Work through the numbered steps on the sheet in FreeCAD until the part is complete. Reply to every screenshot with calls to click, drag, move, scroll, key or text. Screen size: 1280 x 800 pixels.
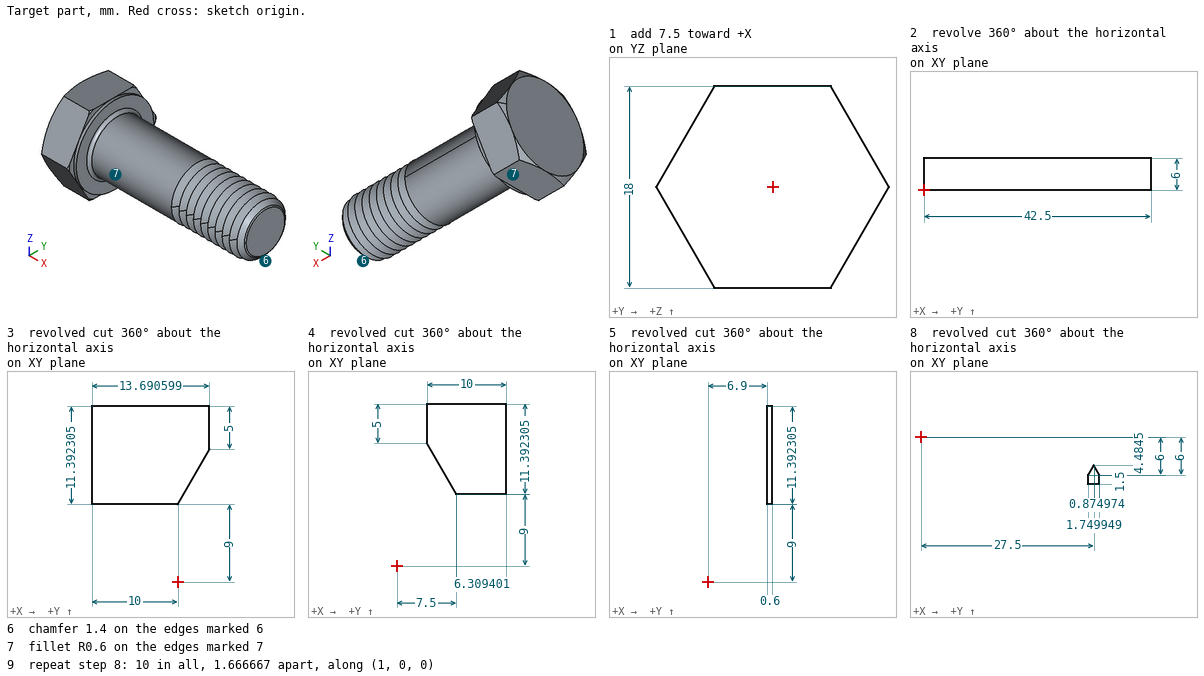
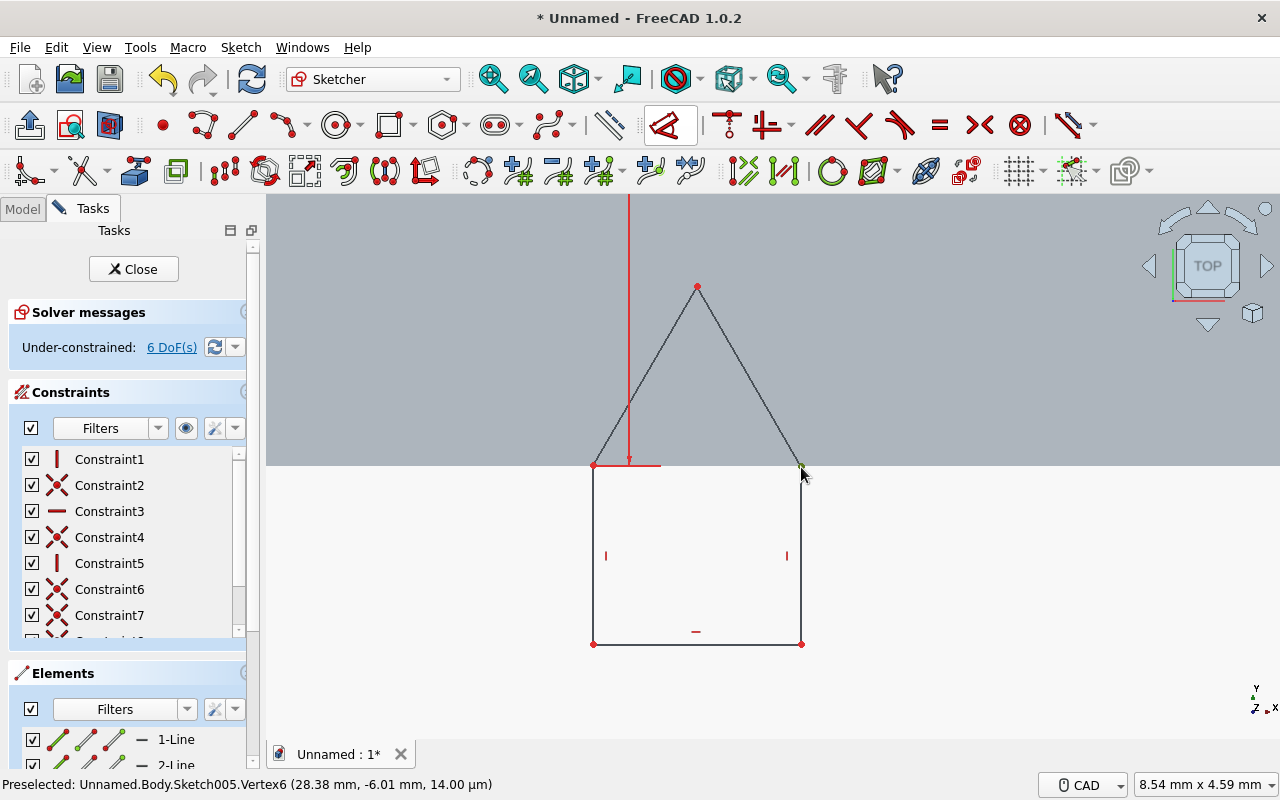
key(i)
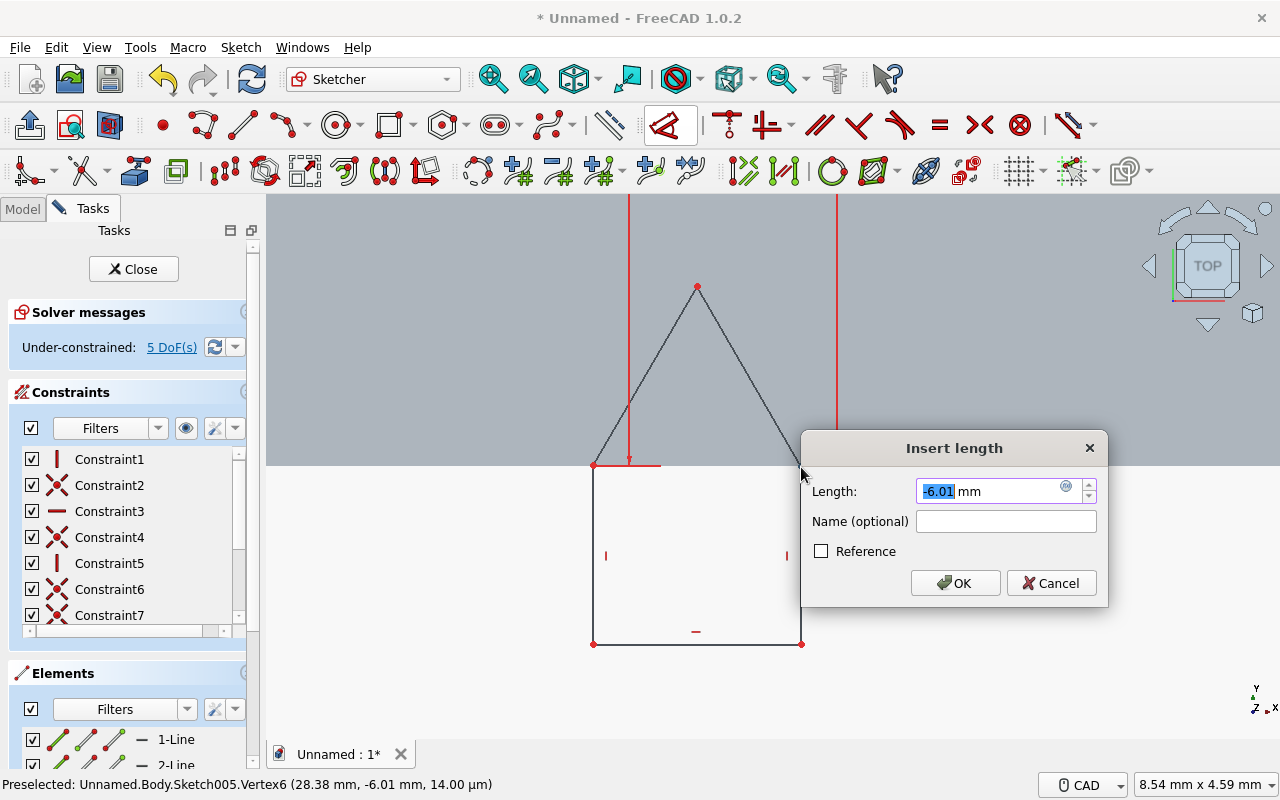
text(-6)
key(Return)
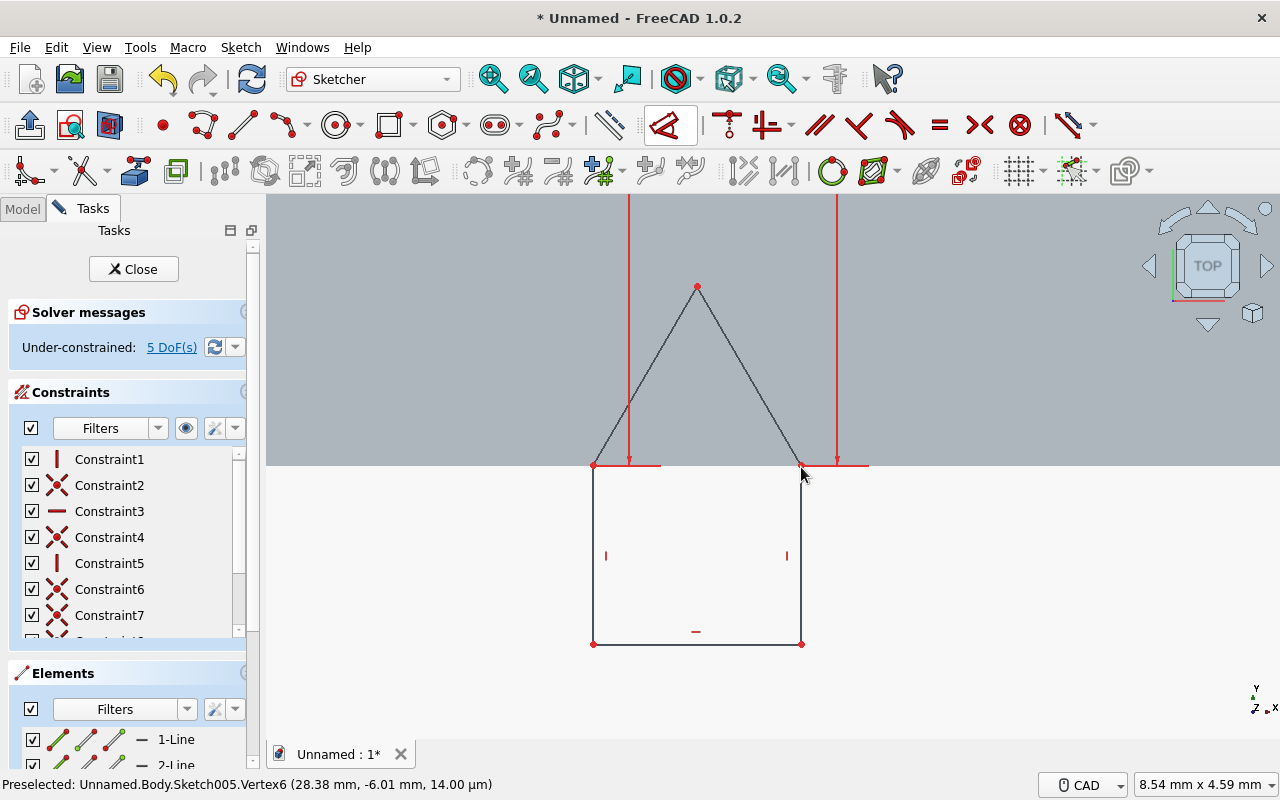
click(593, 519)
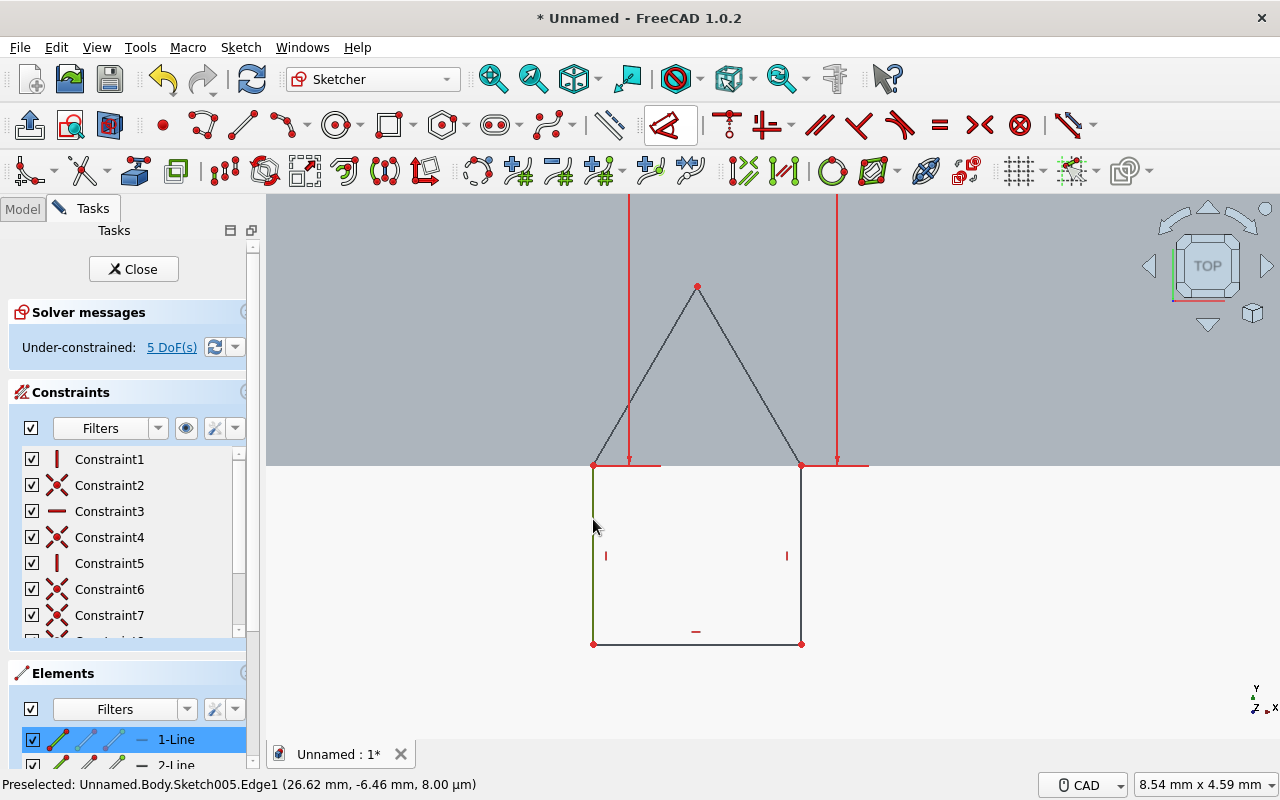
key(i)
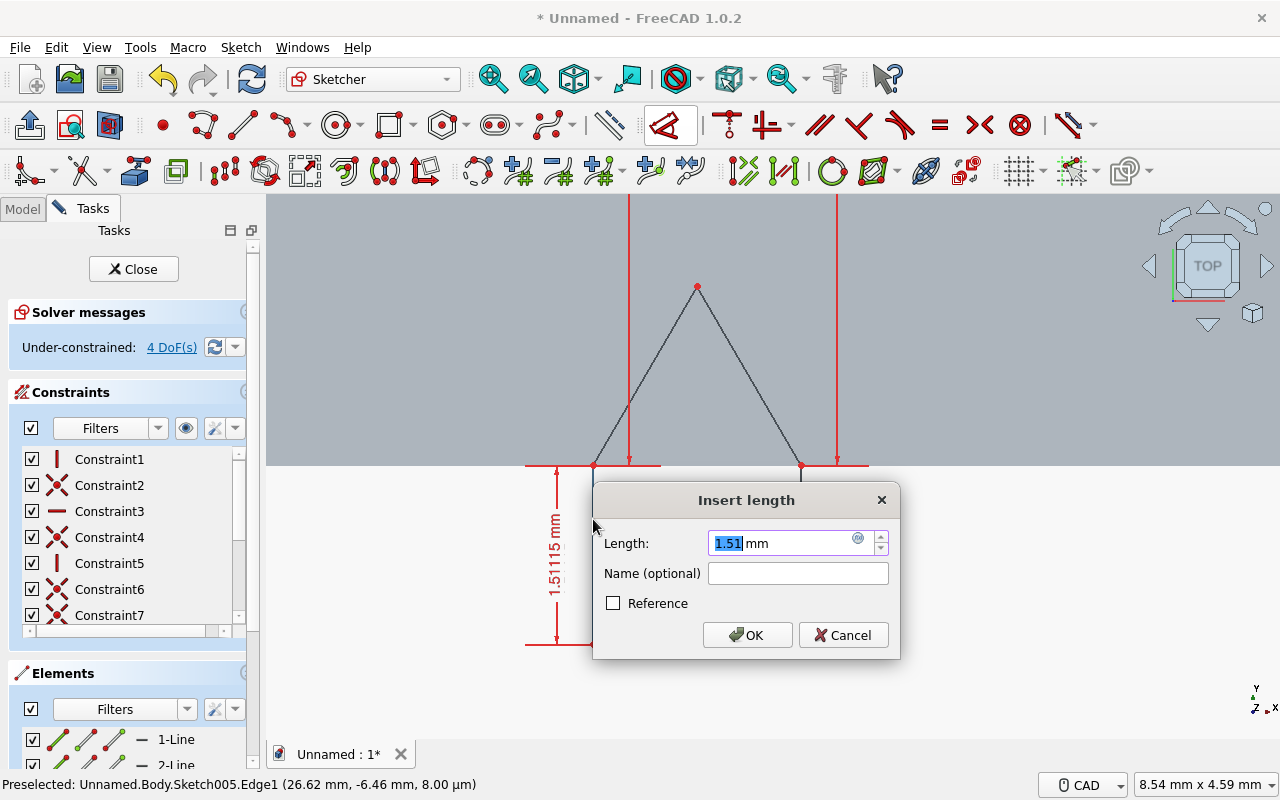
text(1.5)
key(Return)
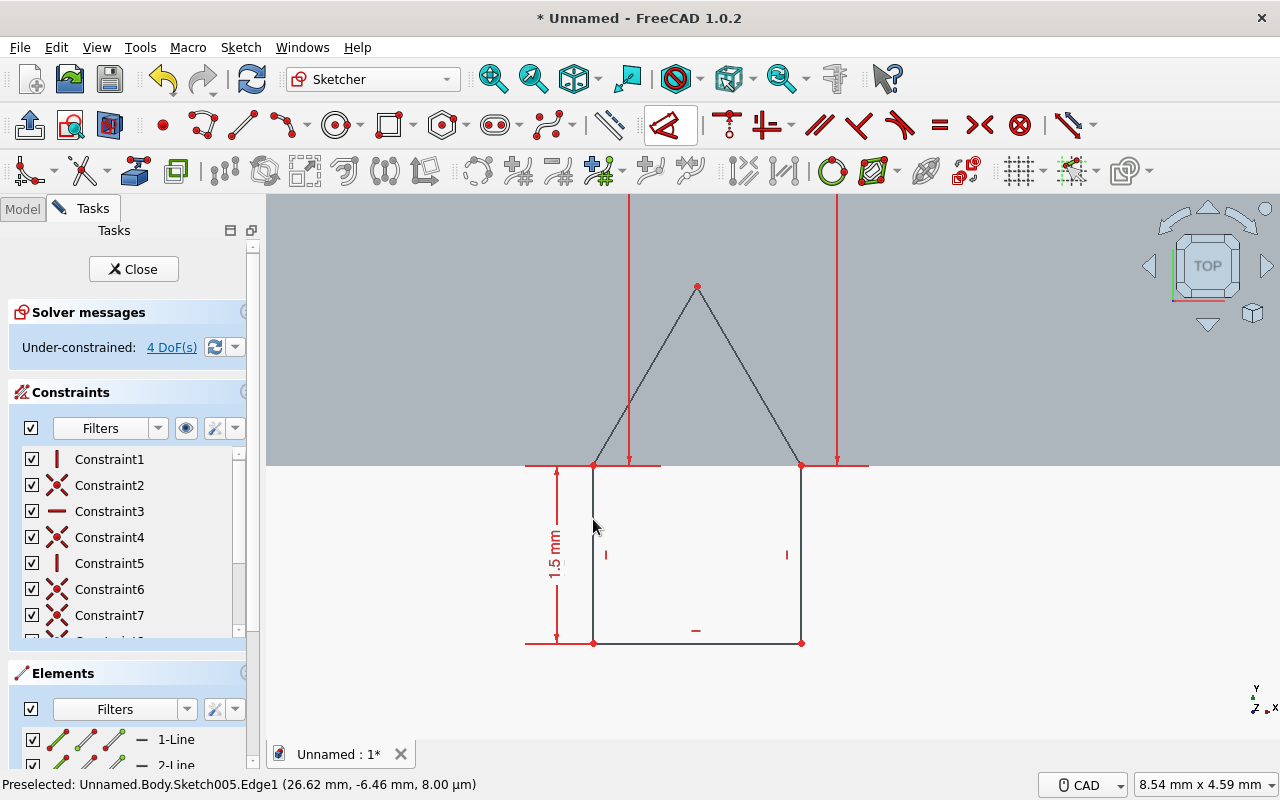
click(697, 287)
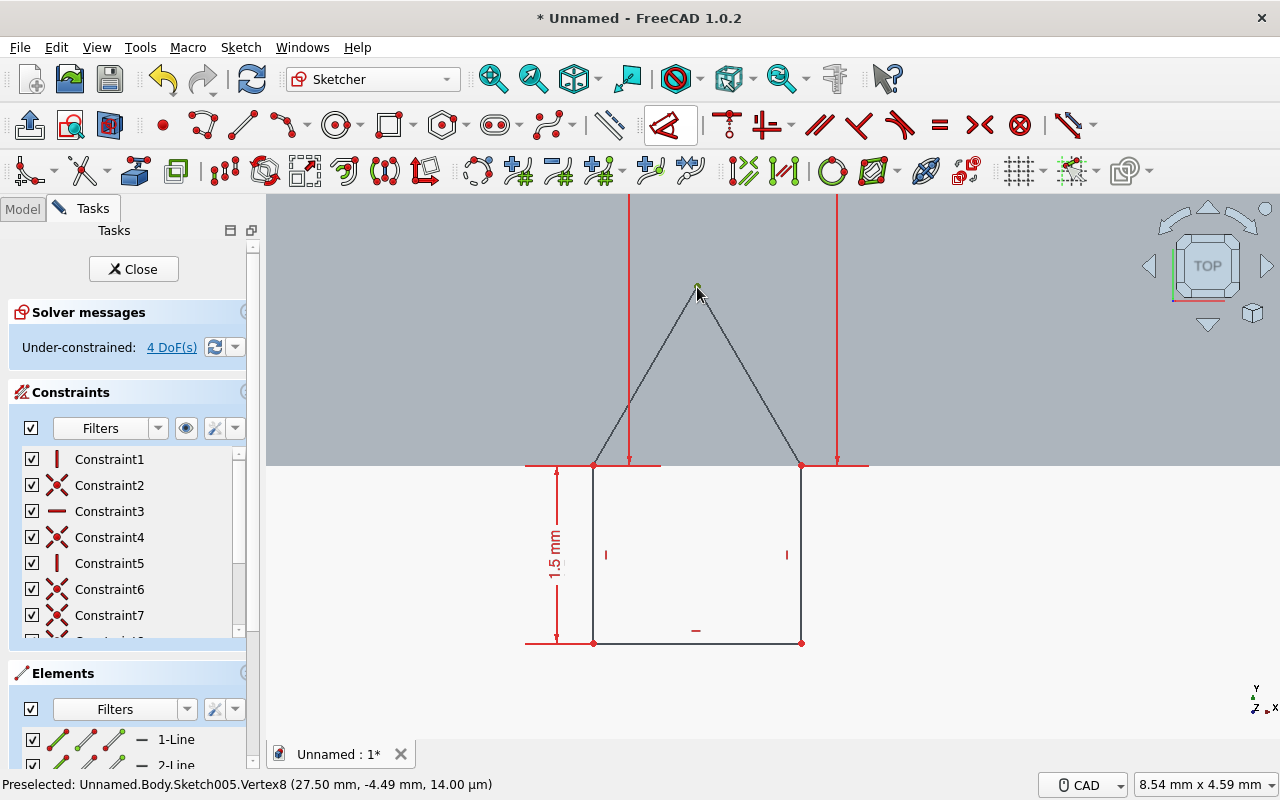
click(692, 126)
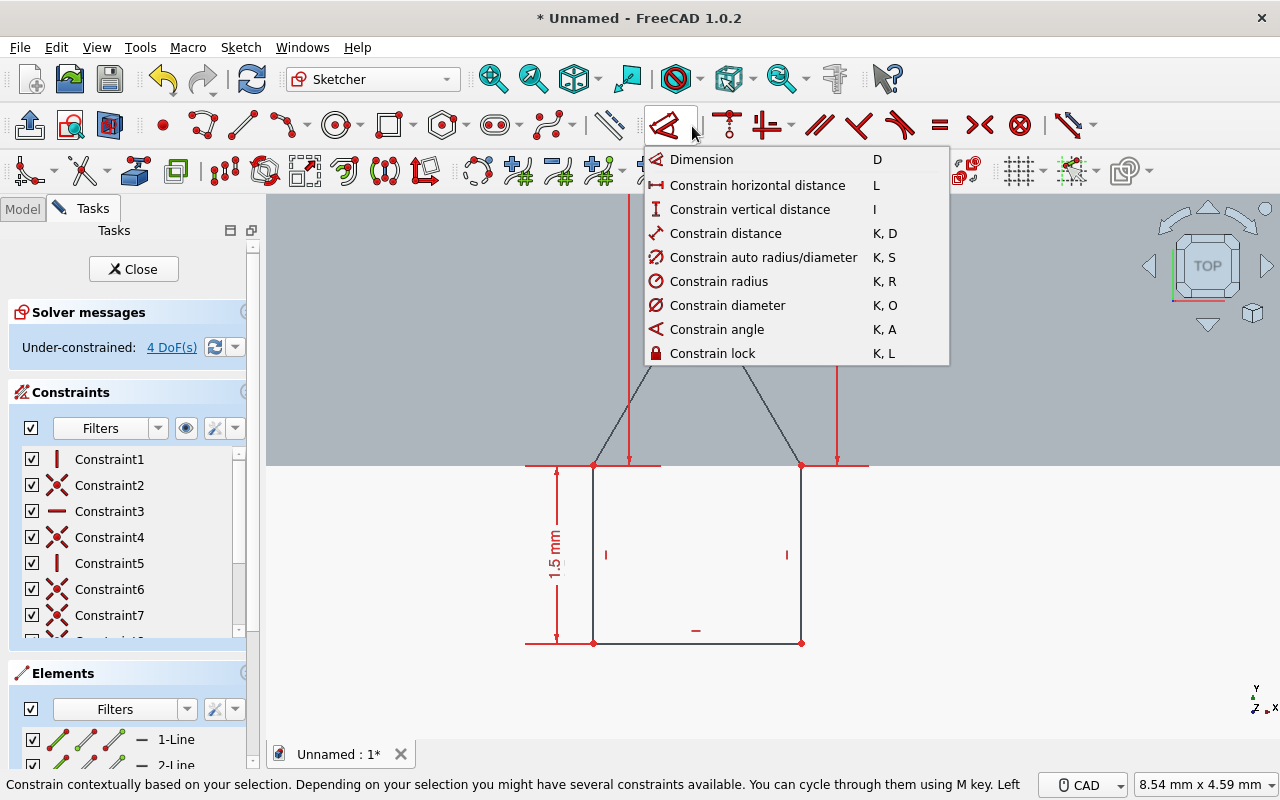
click(797, 185)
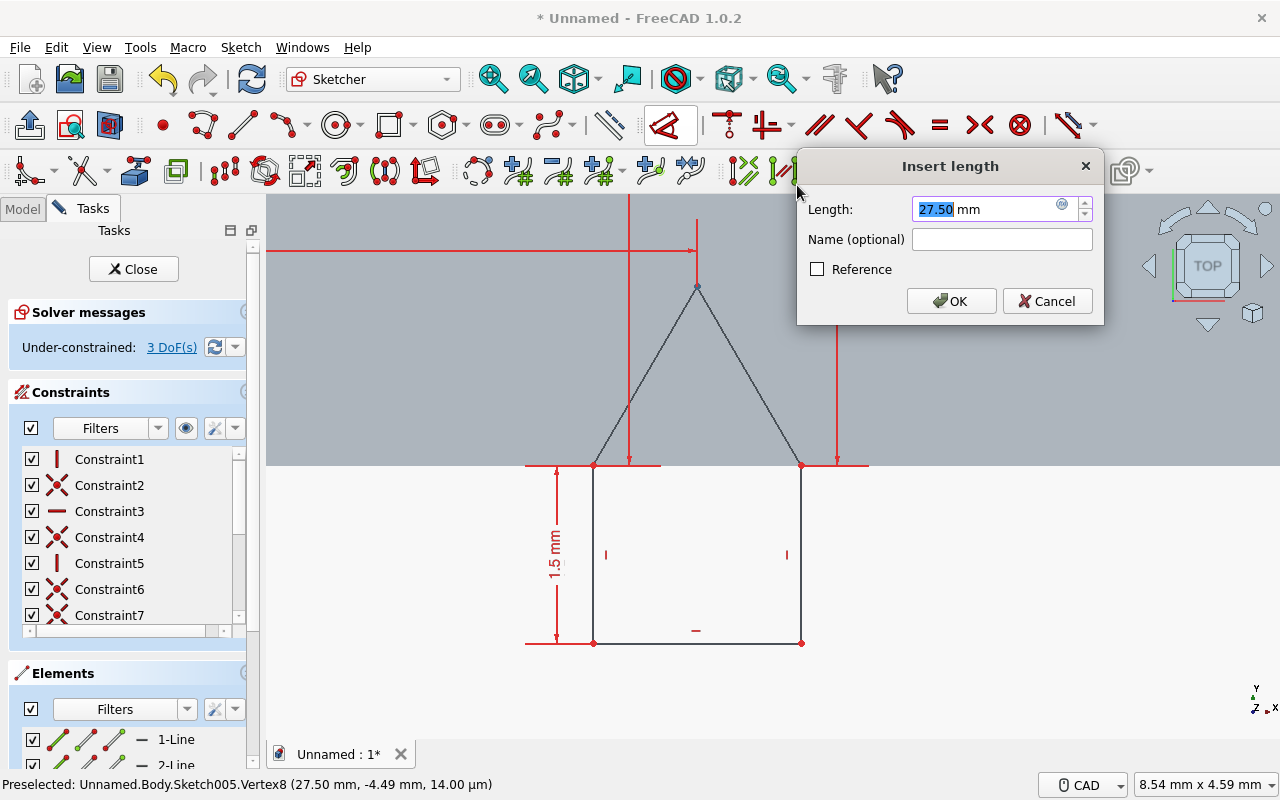
text(27.5)
key(Return)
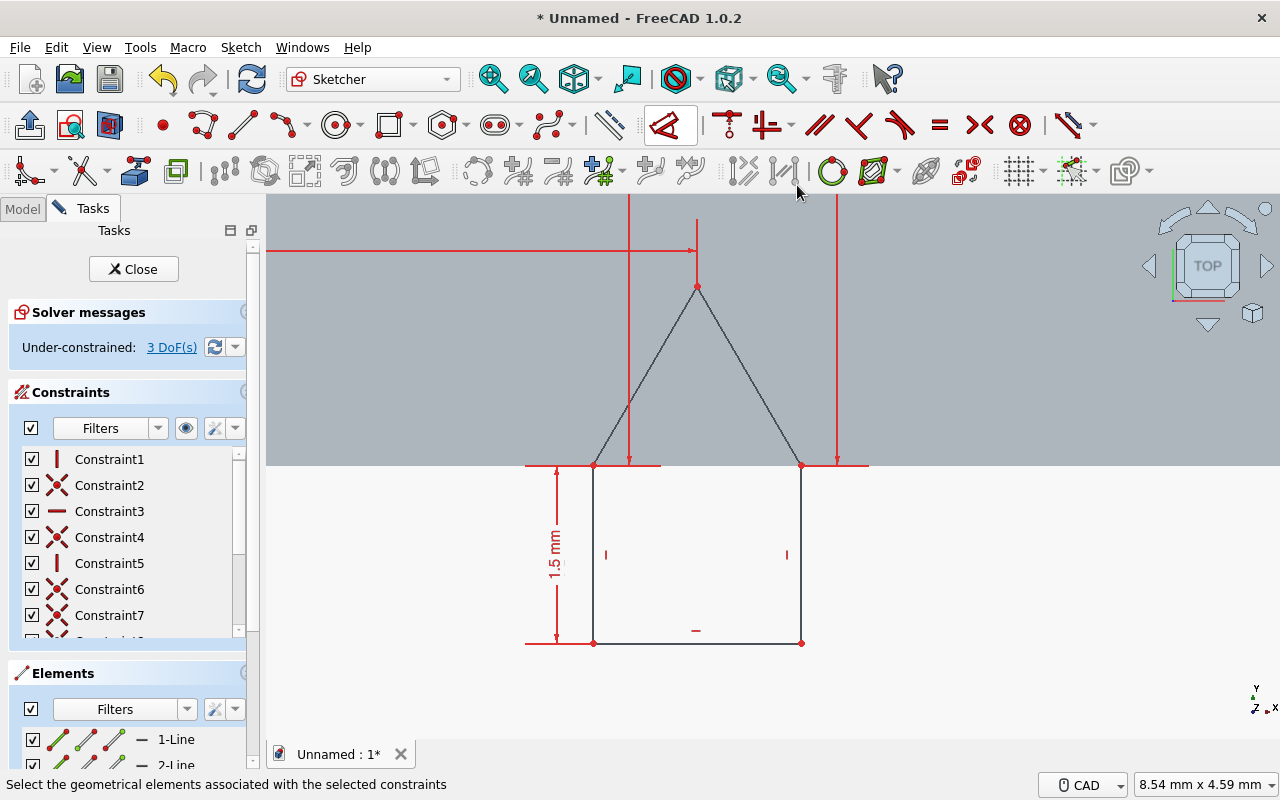
click(697, 287)